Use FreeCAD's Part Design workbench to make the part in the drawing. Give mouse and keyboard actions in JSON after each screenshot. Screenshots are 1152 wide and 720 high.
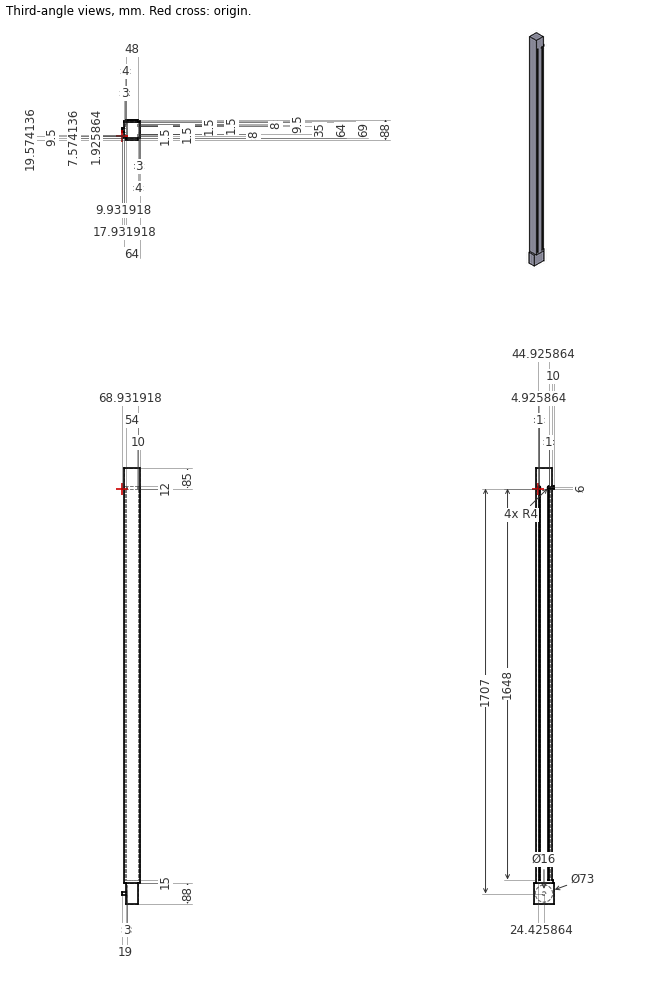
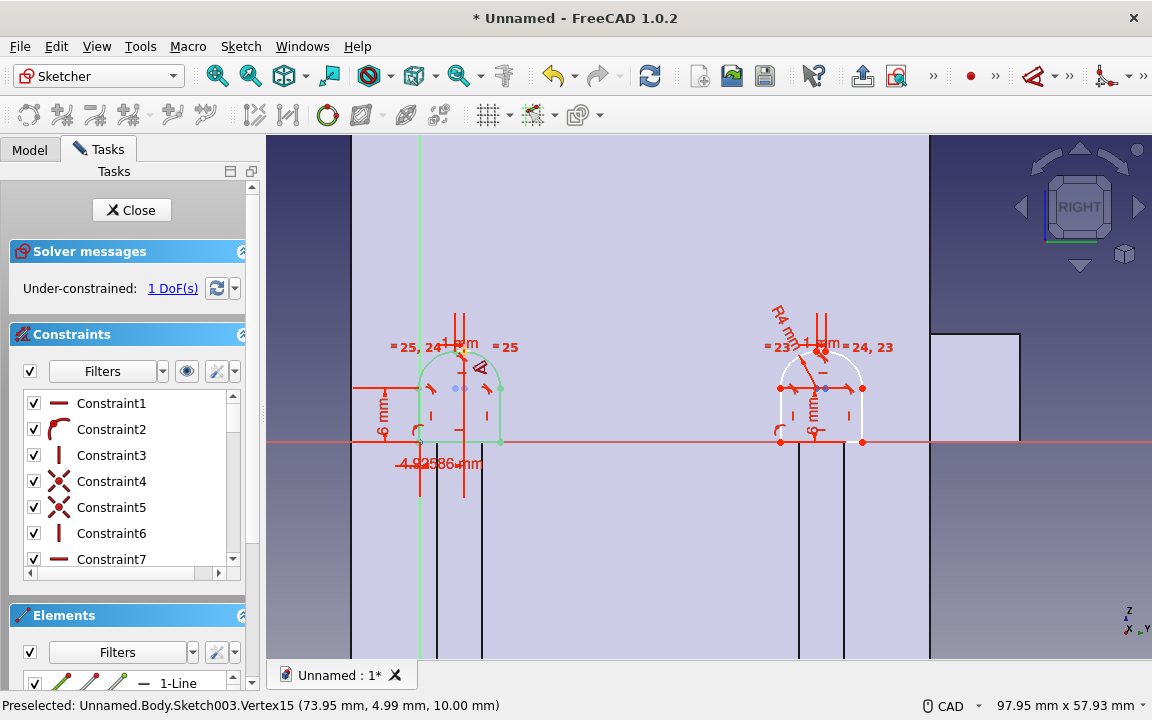
{"action": "scroll", "coordinate": [826, 352], "scroll_direction": "up", "scroll_amount": 2}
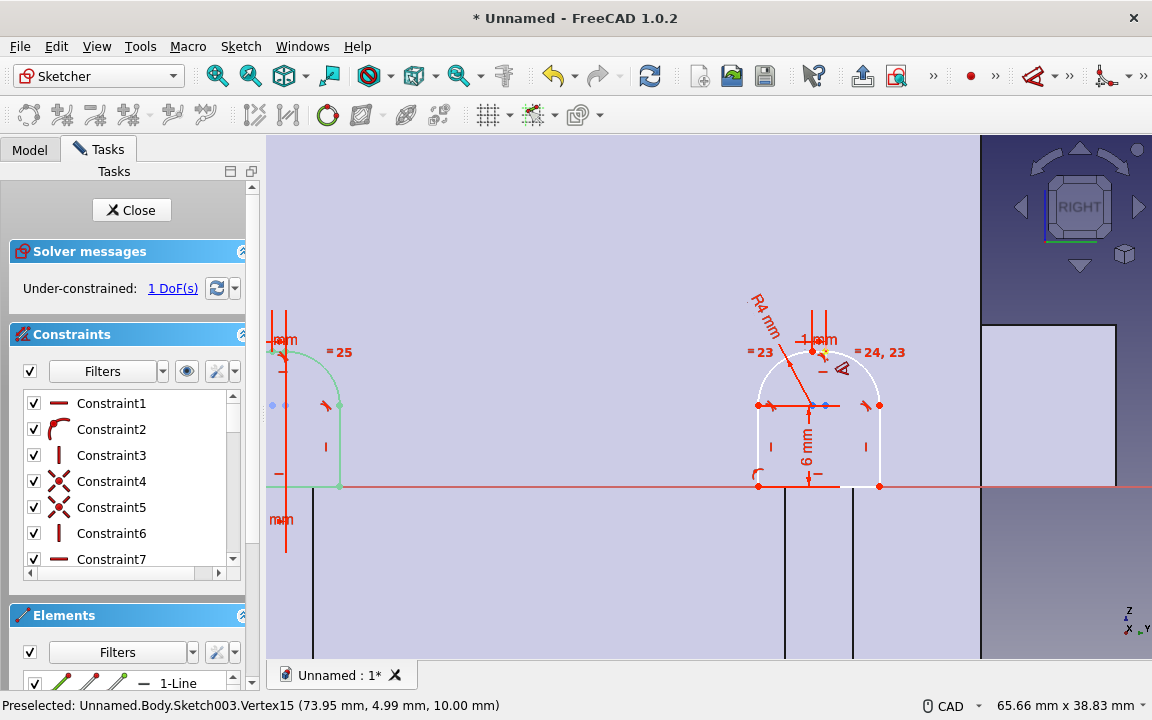
{"action": "left_click", "coordinate": [826, 352]}
{"action": "left_click", "coordinate": [560, 521]}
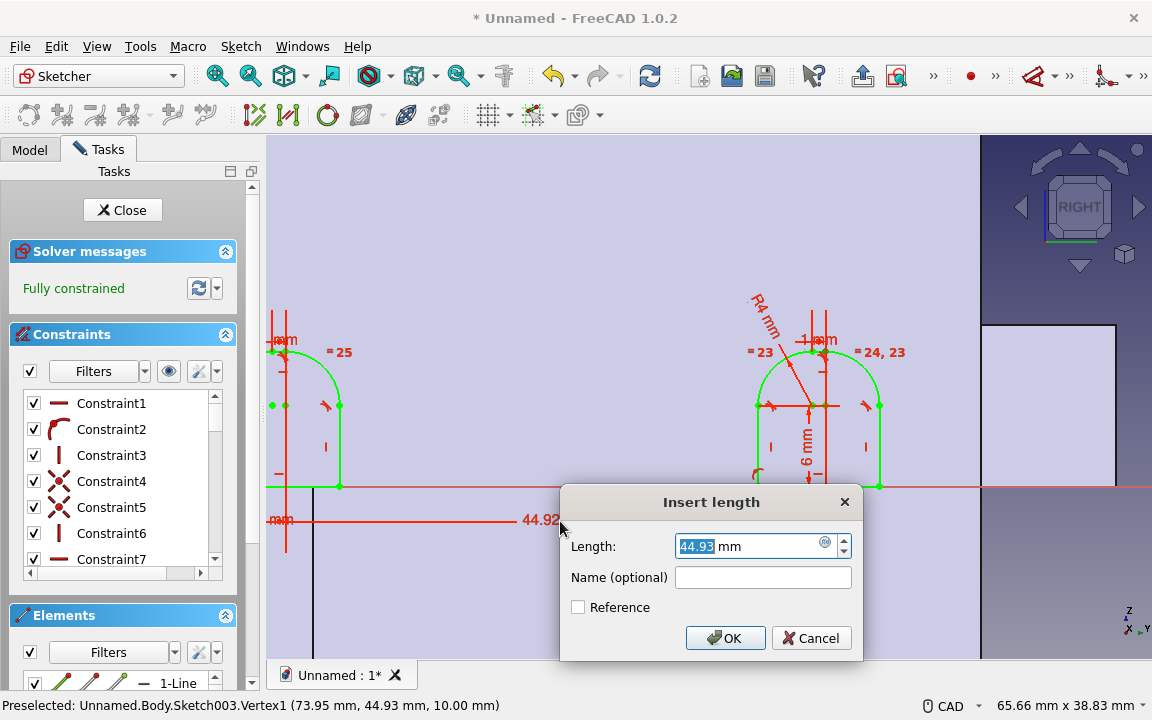
{"action": "type", "text": "44.925864"}
{"action": "key", "text": "Return"}
{"action": "key", "text": "Escape"}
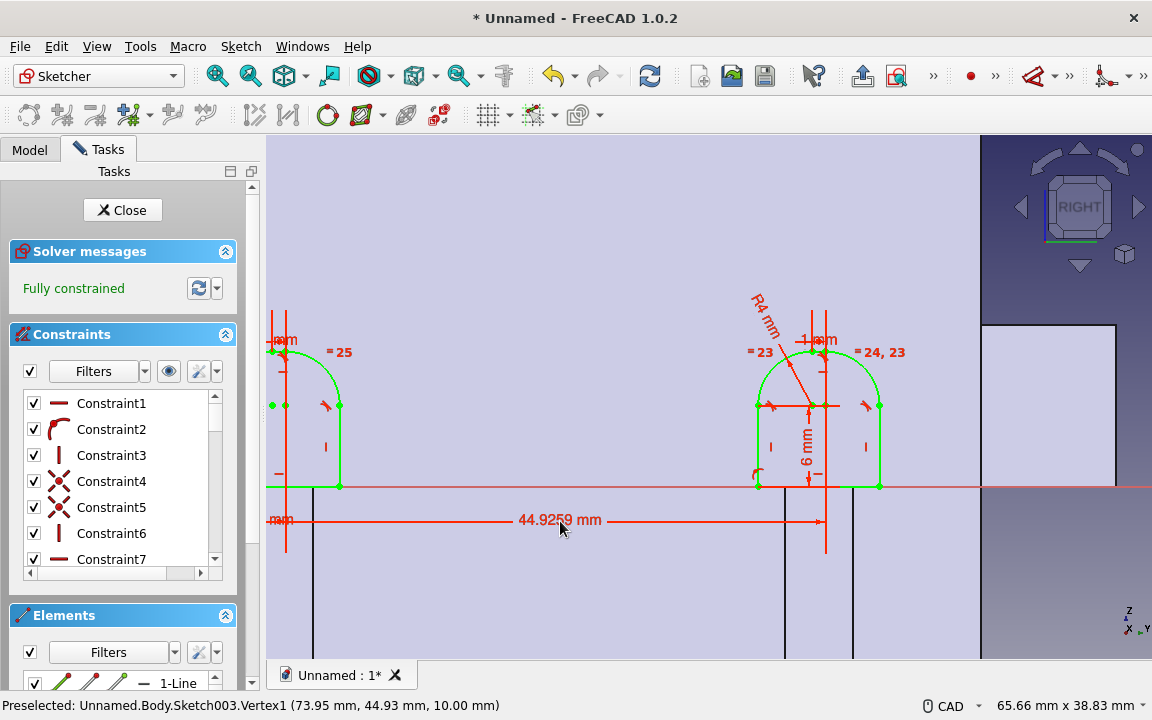
{"action": "left_click", "coordinate": [123, 210]}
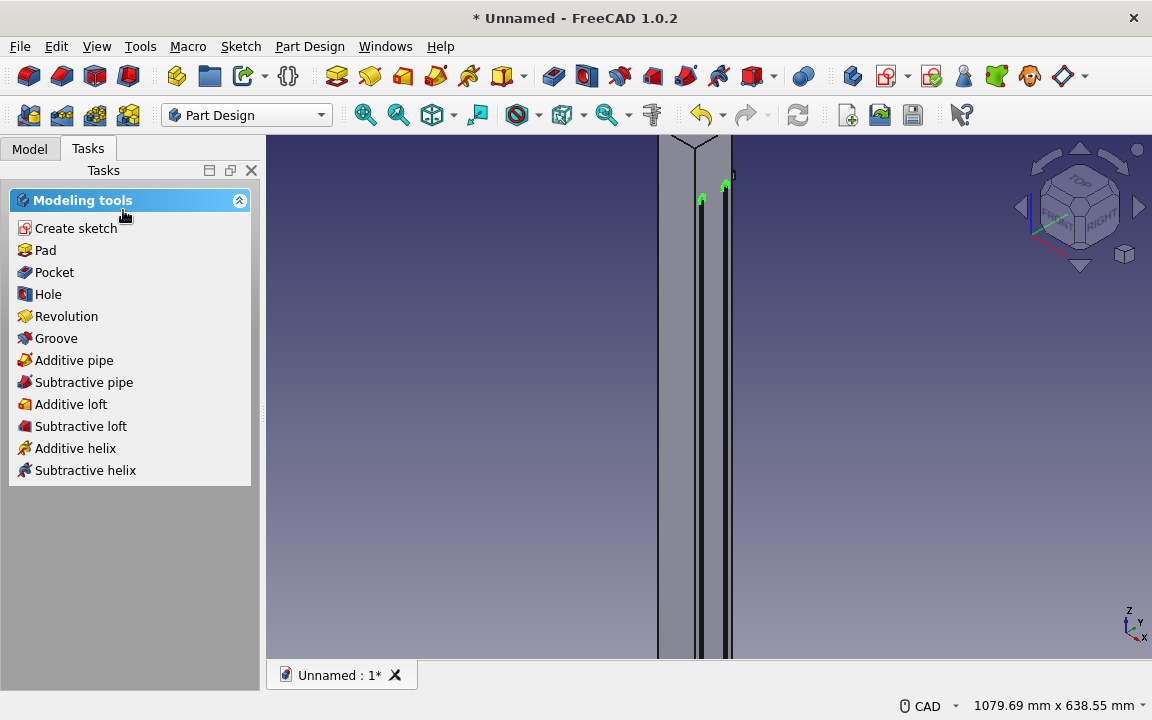
{"action": "left_click", "coordinate": [554, 76]}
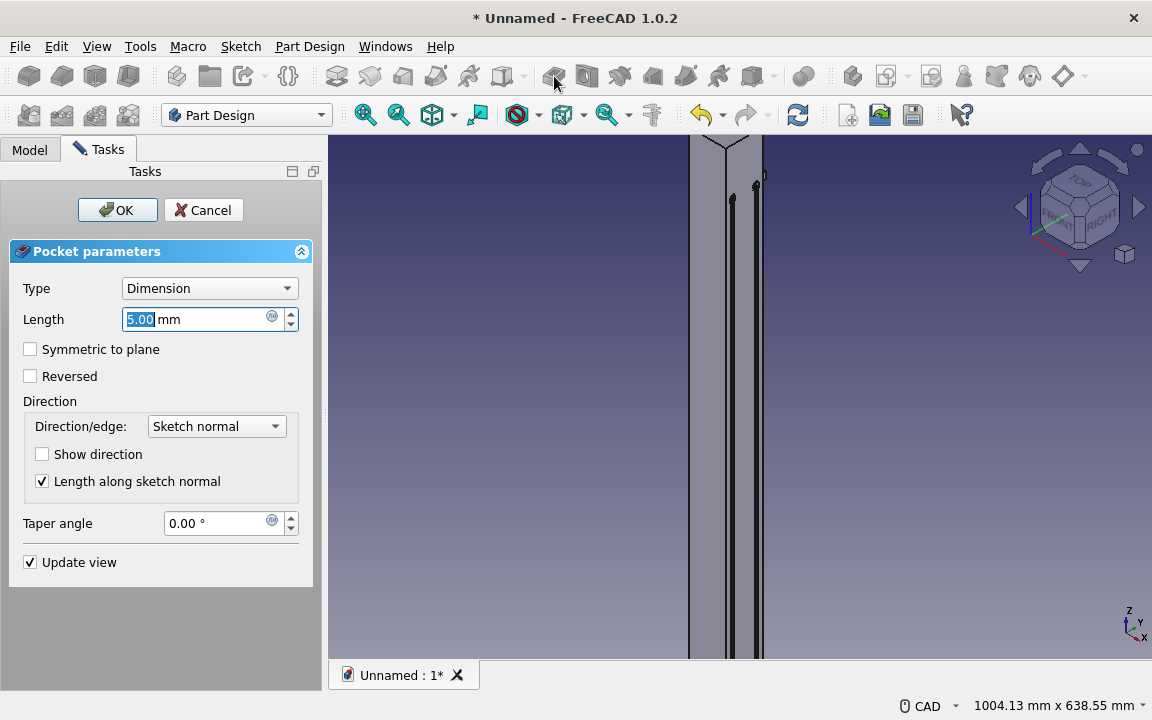
{"action": "type", "text": "10"}
{"action": "key", "text": "Tab"}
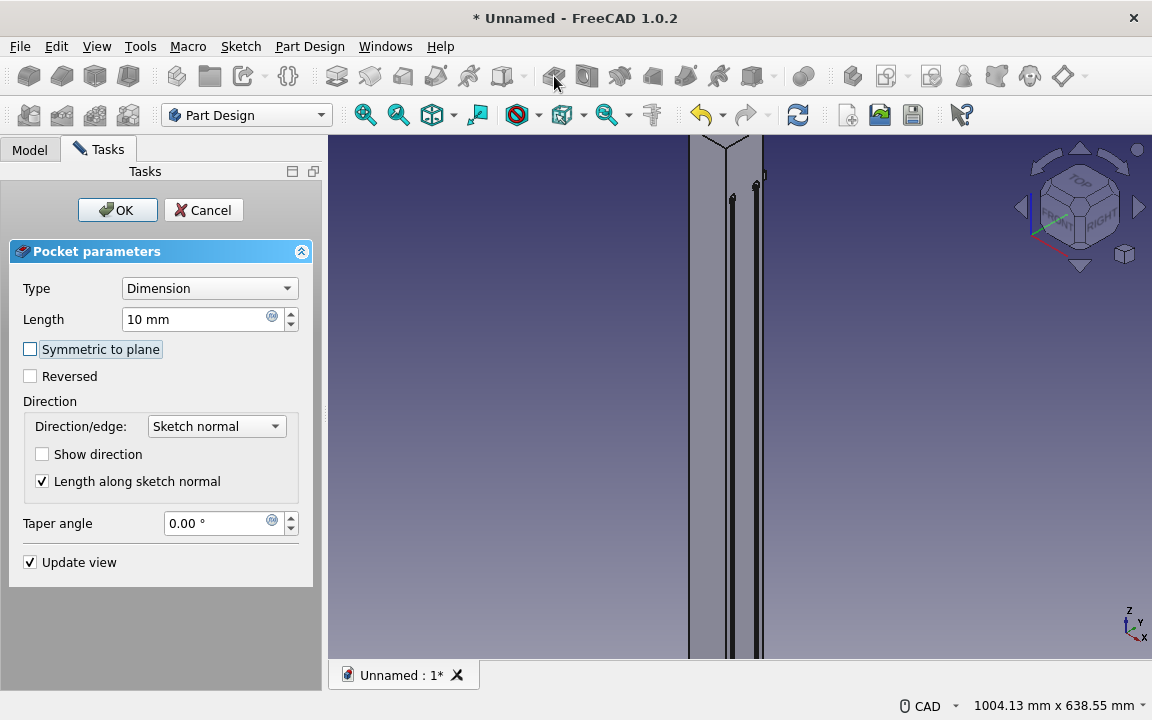
{"action": "left_click", "coordinate": [118, 210]}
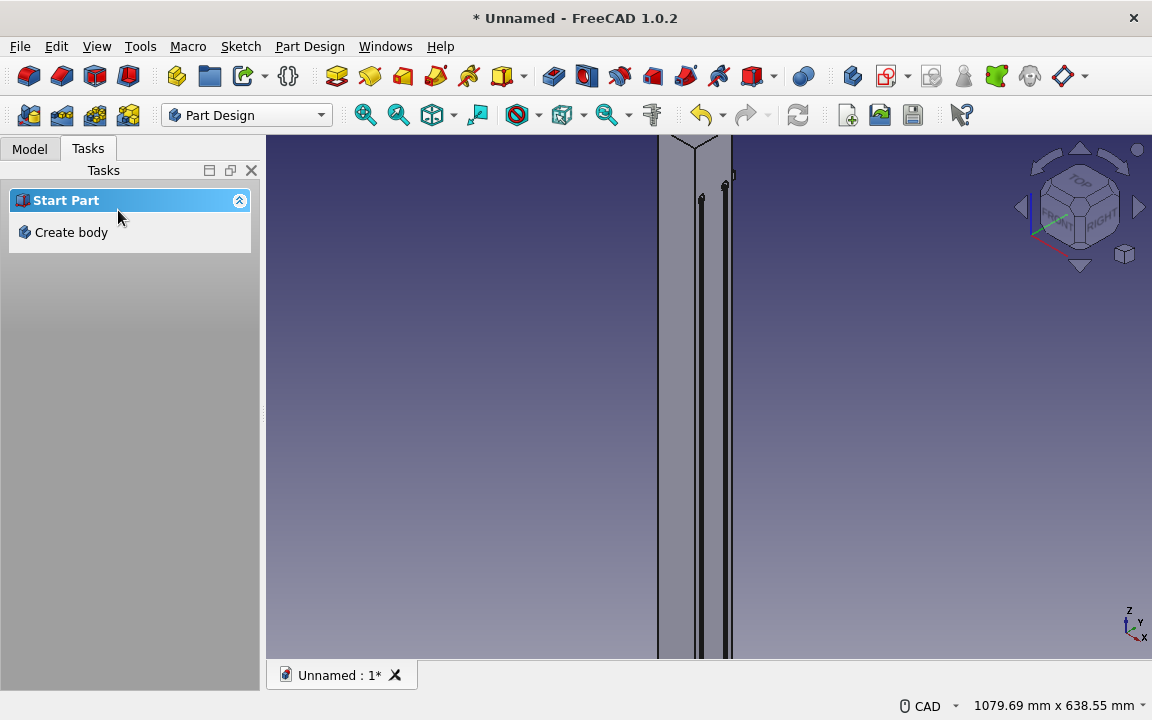
{"action": "left_click", "coordinate": [366, 116]}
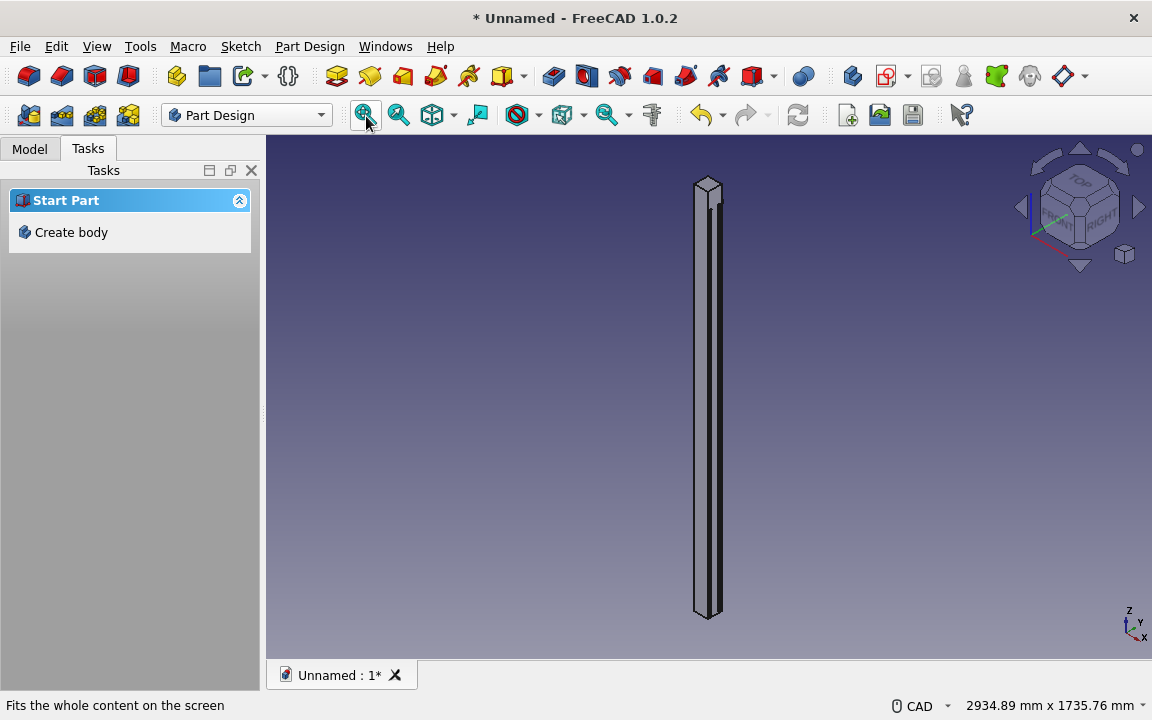
{"action": "left_click", "coordinate": [30, 148]}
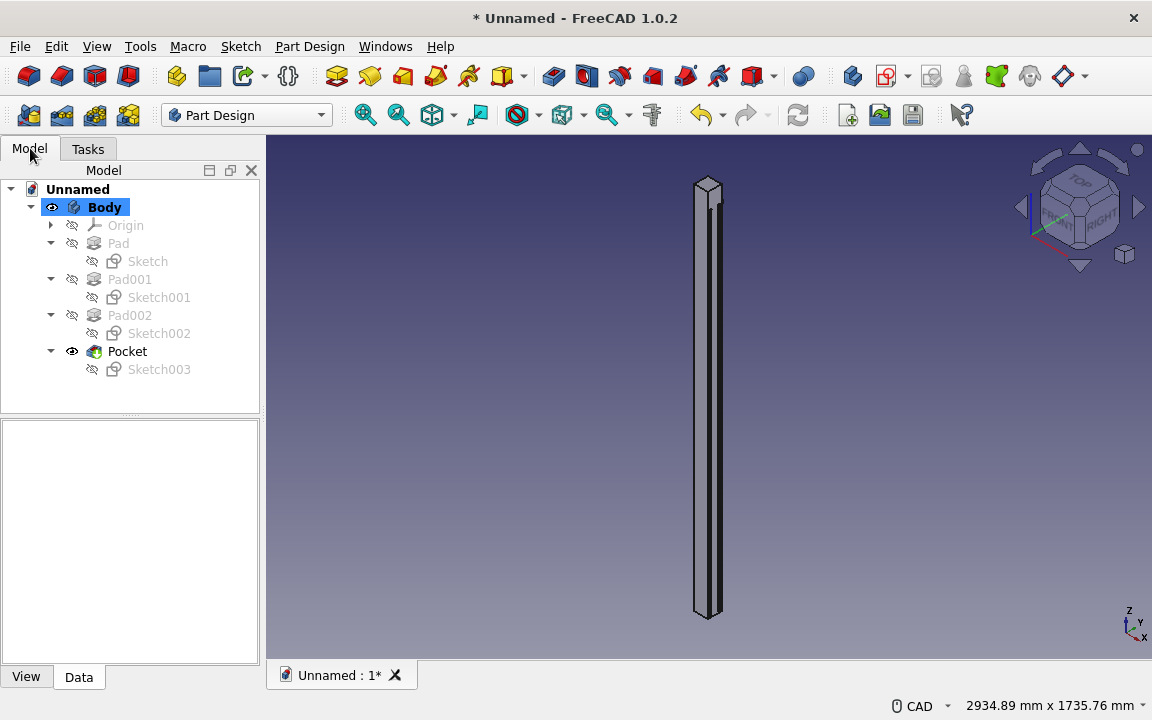
{"action": "left_click", "coordinate": [51, 225]}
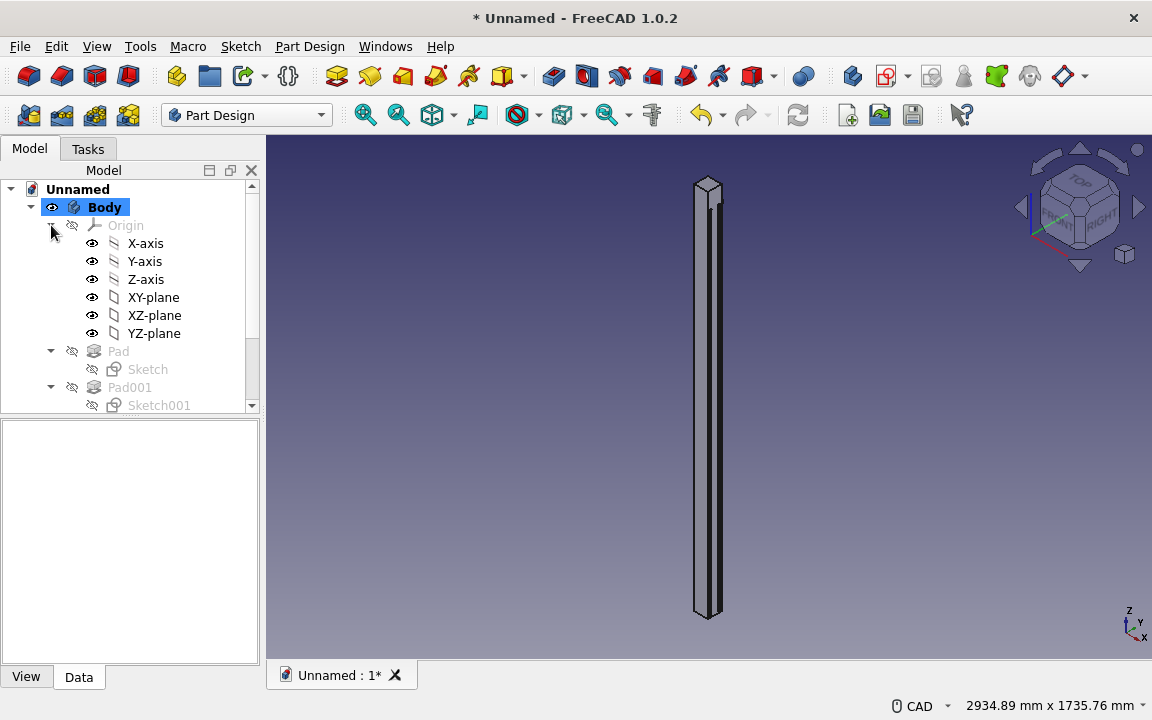
{"action": "left_click", "coordinate": [137, 333]}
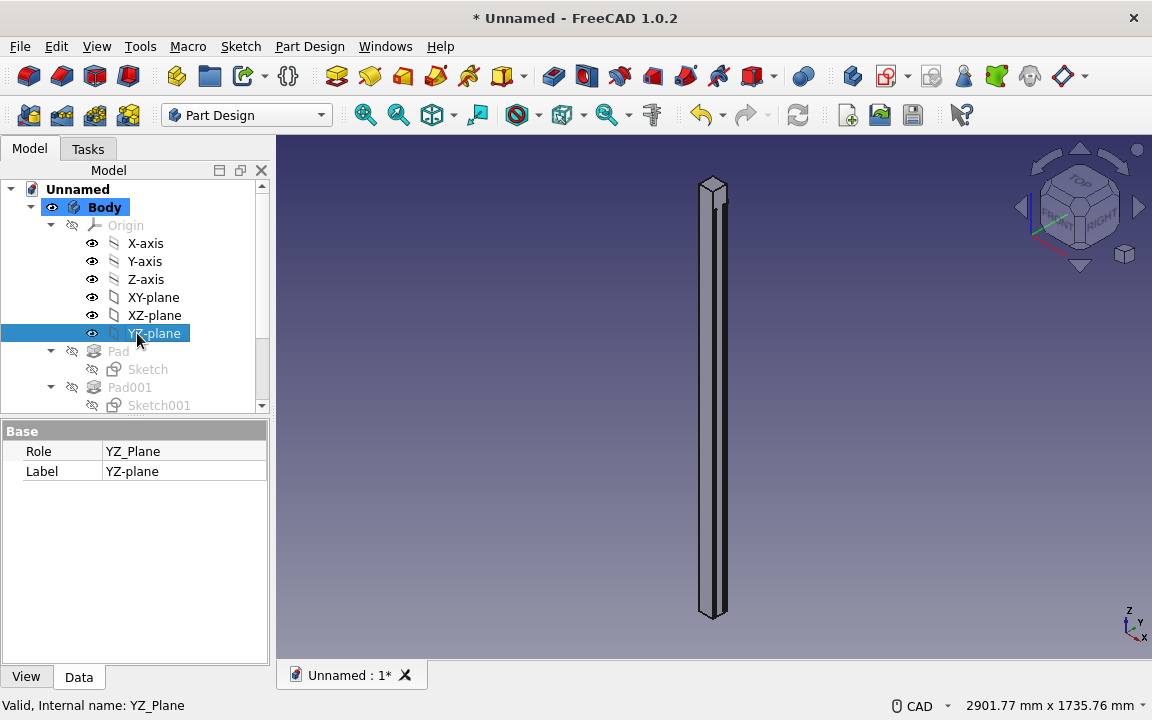
{"action": "left_click", "coordinate": [1062, 76]}